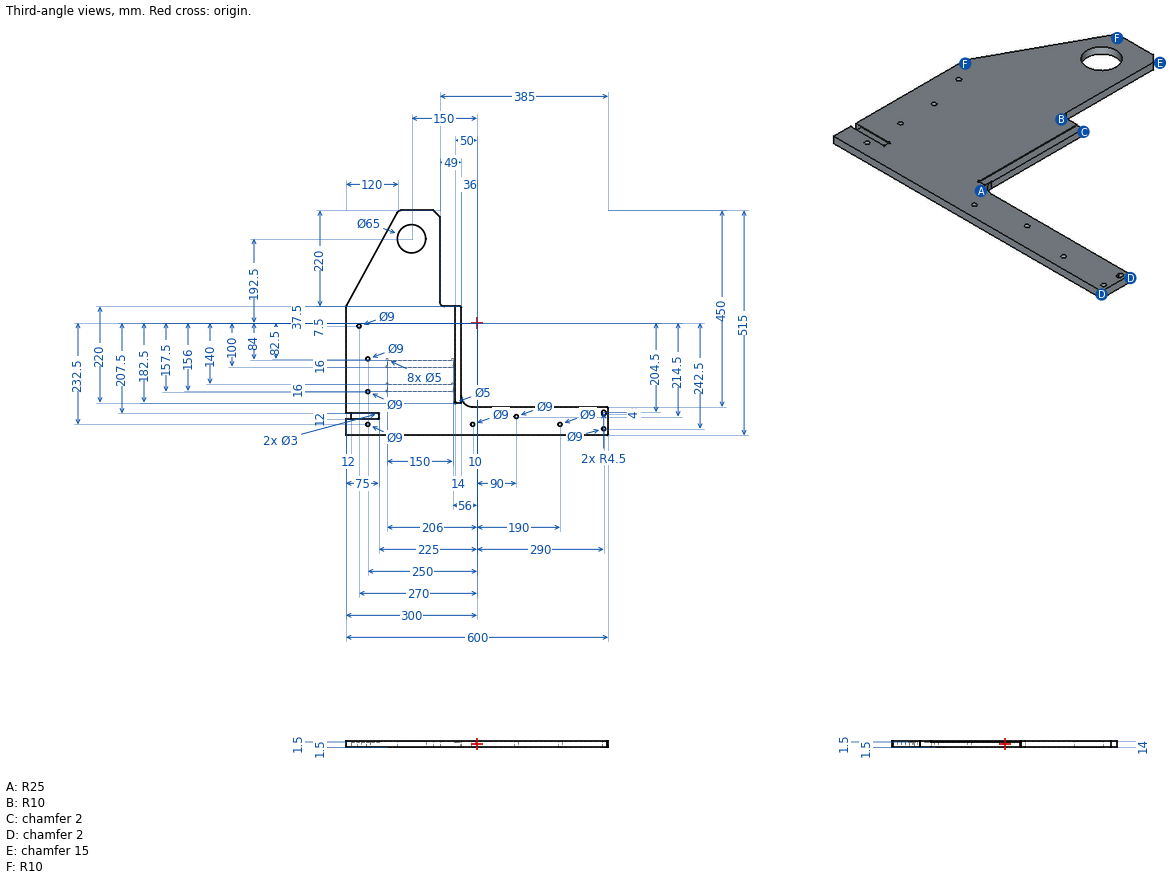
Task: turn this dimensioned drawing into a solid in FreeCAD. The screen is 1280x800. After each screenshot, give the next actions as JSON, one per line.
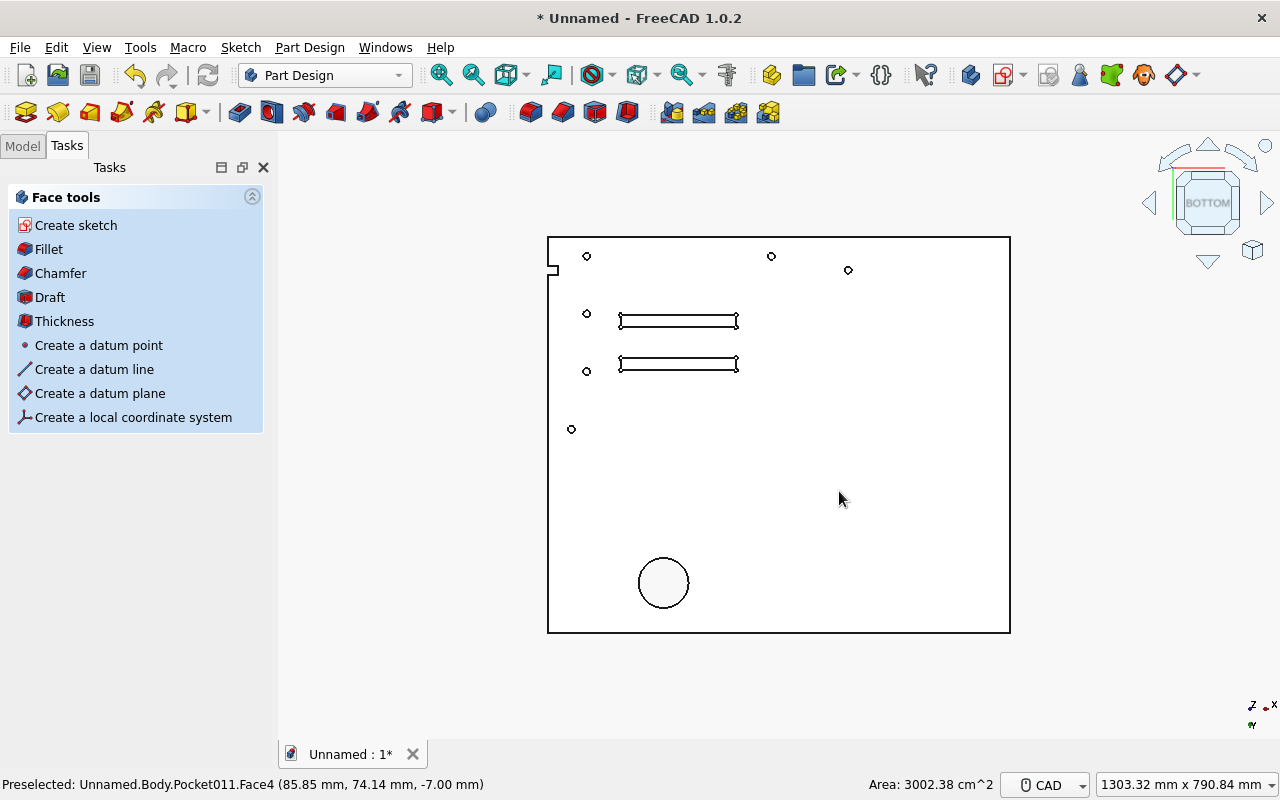
{"action": "left_click", "coordinate": [1004, 76]}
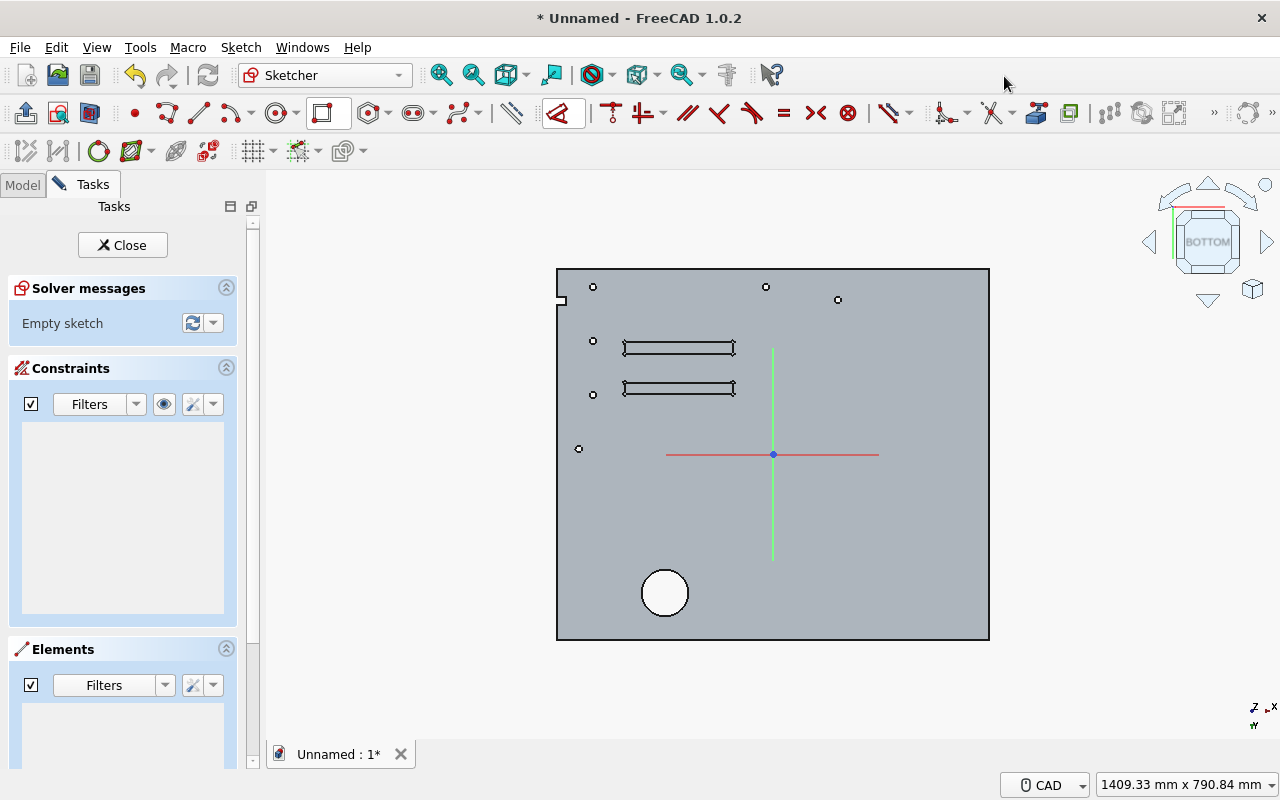
{"action": "scroll", "coordinate": [920, 278], "scroll_direction": "up", "scroll_amount": 15}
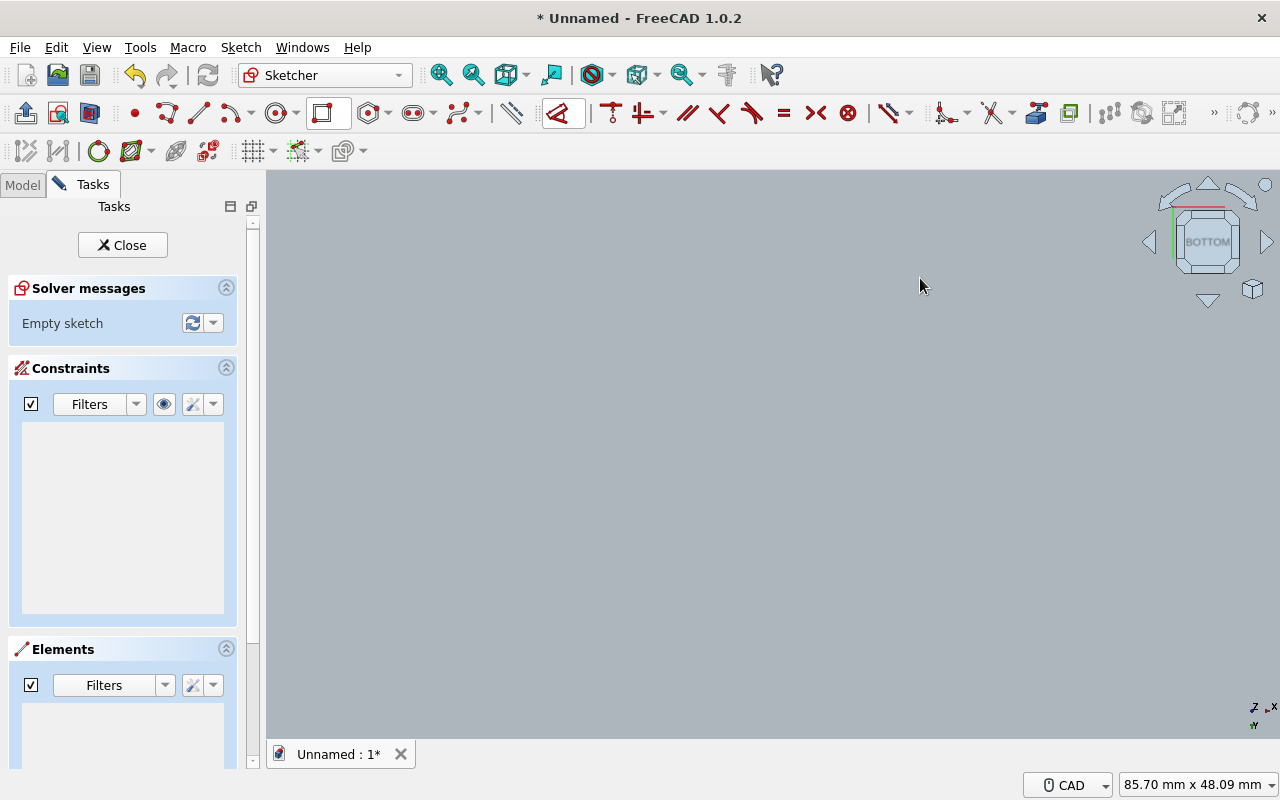
{"action": "scroll", "coordinate": [699, 462], "scroll_direction": "up", "scroll_amount": 5}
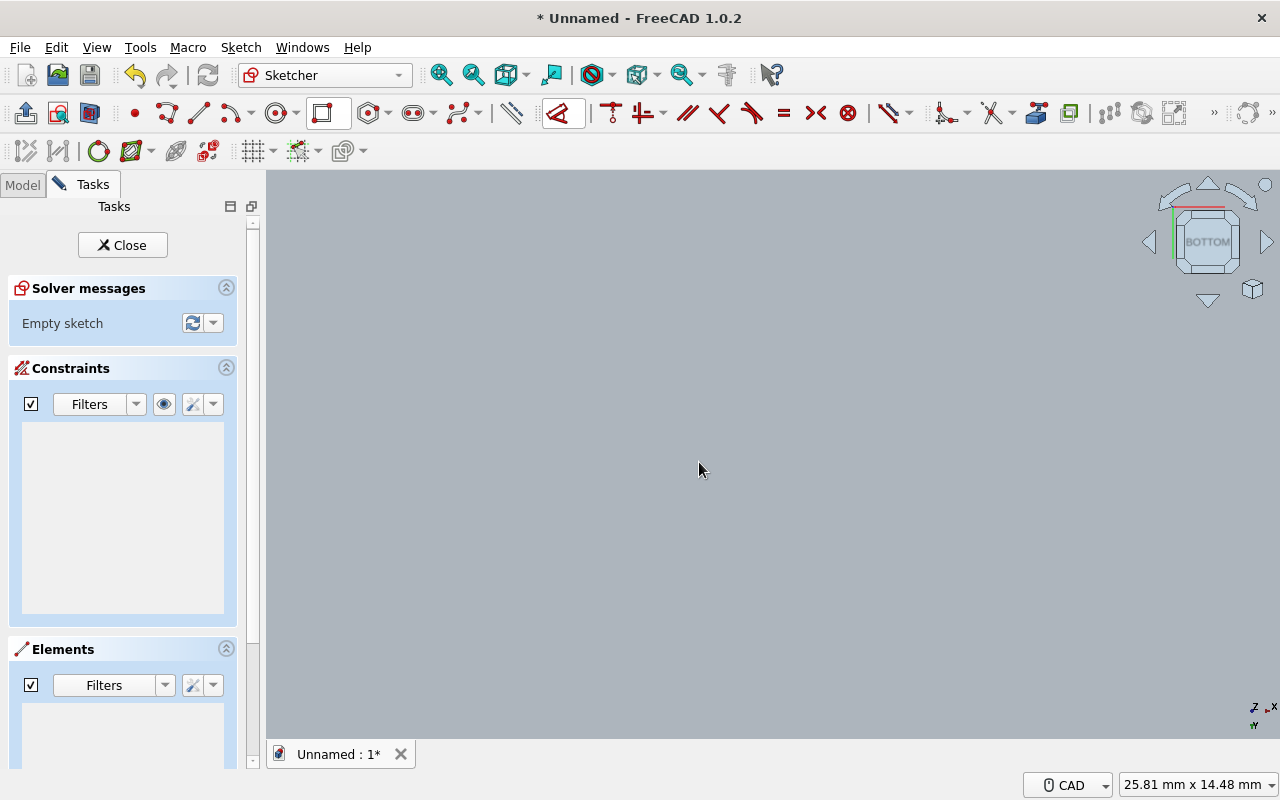
{"action": "left_click", "coordinate": [276, 114]}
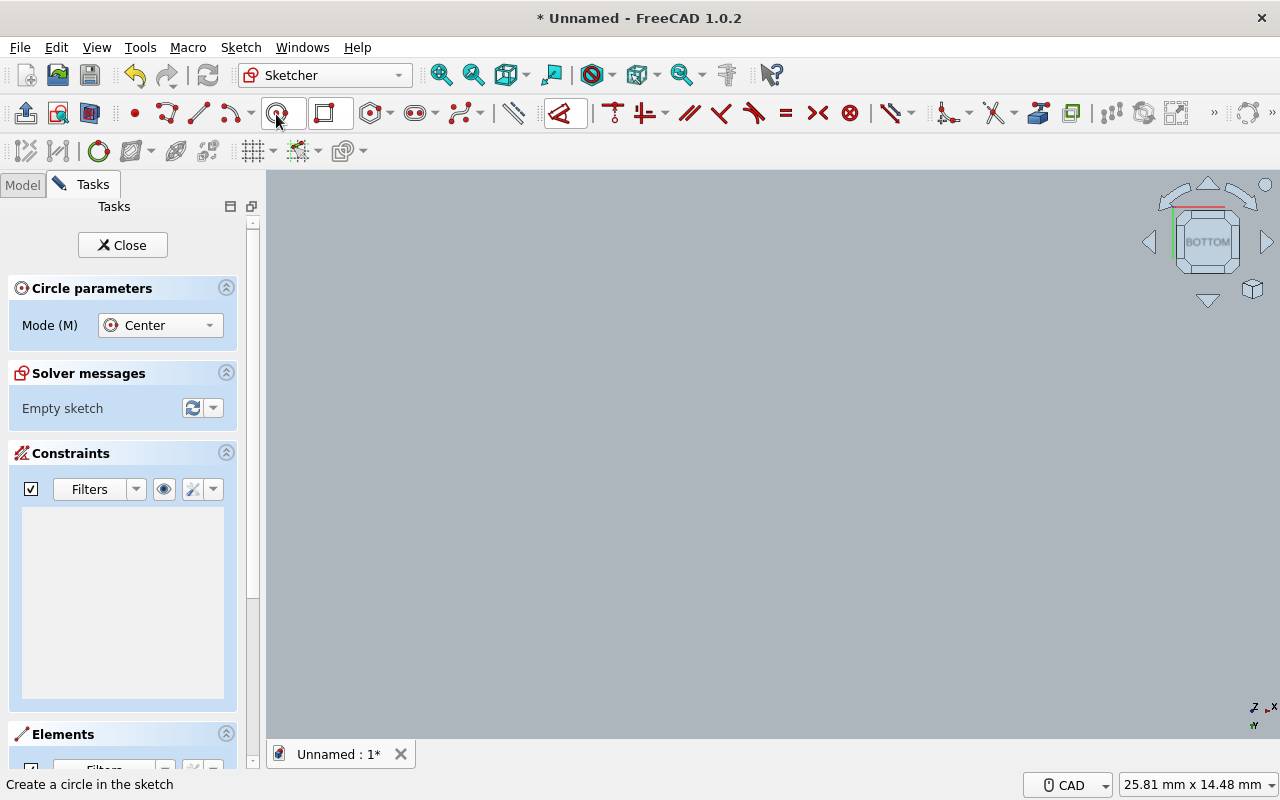
{"action": "left_click", "coordinate": [703, 454]}
{"action": "mouse_move", "coordinate": [828, 329]}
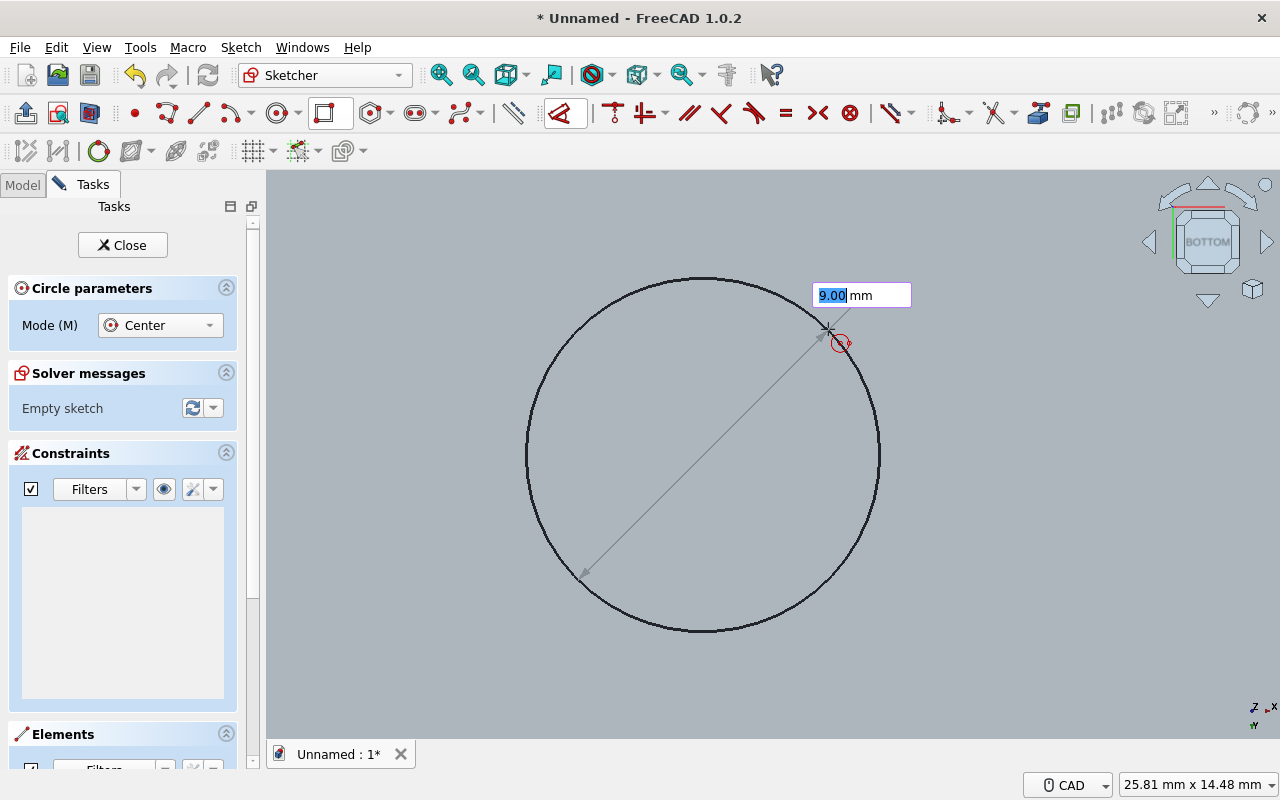
{"action": "type", "text": "9"}
{"action": "key", "text": "Return"}
{"action": "key", "text": "Escape"}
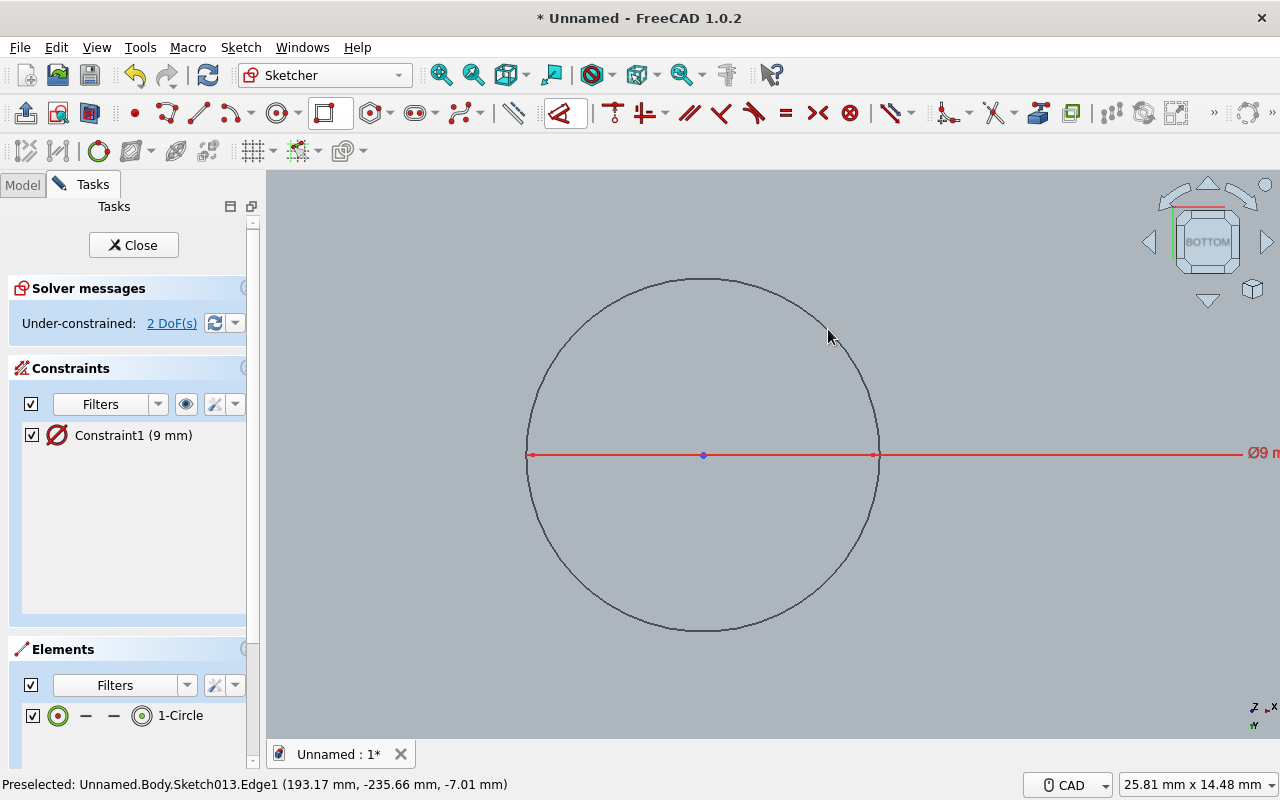
{"action": "left_click", "coordinate": [703, 455]}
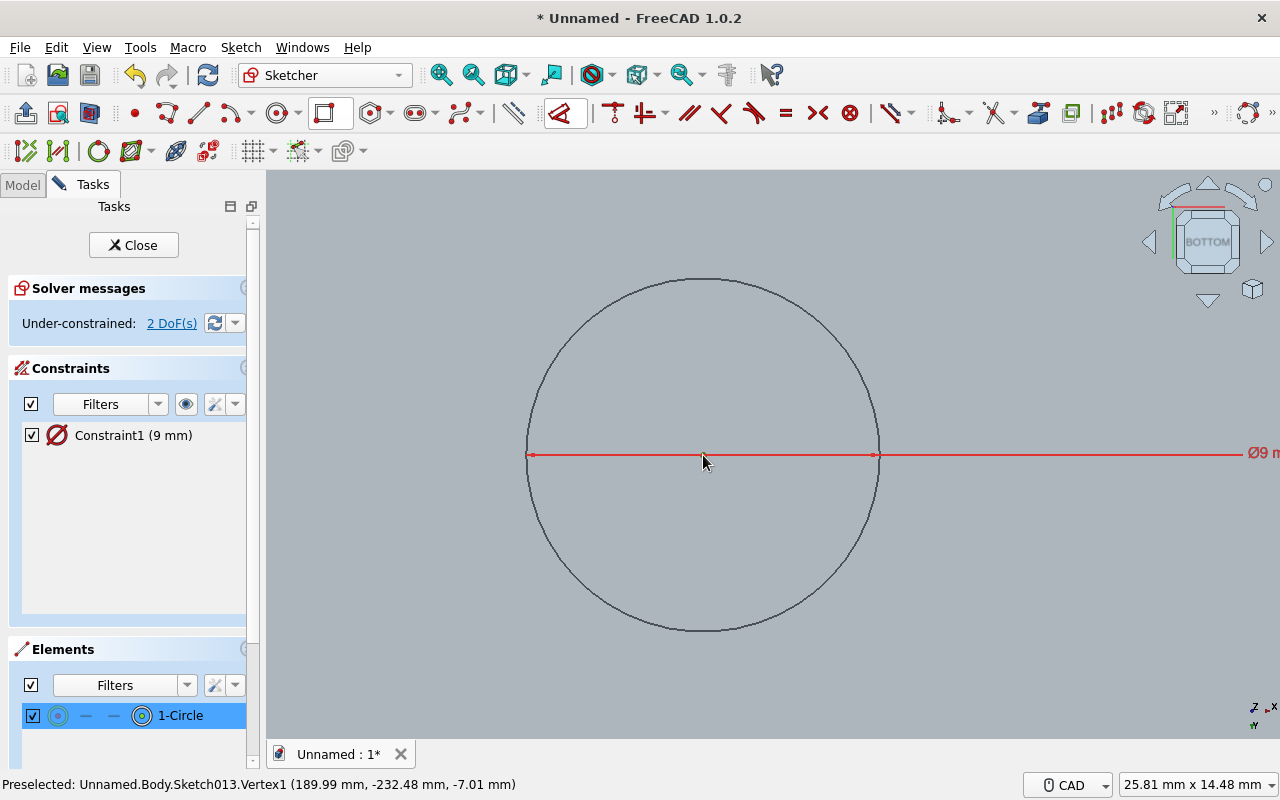
{"action": "left_click", "coordinate": [582, 114]}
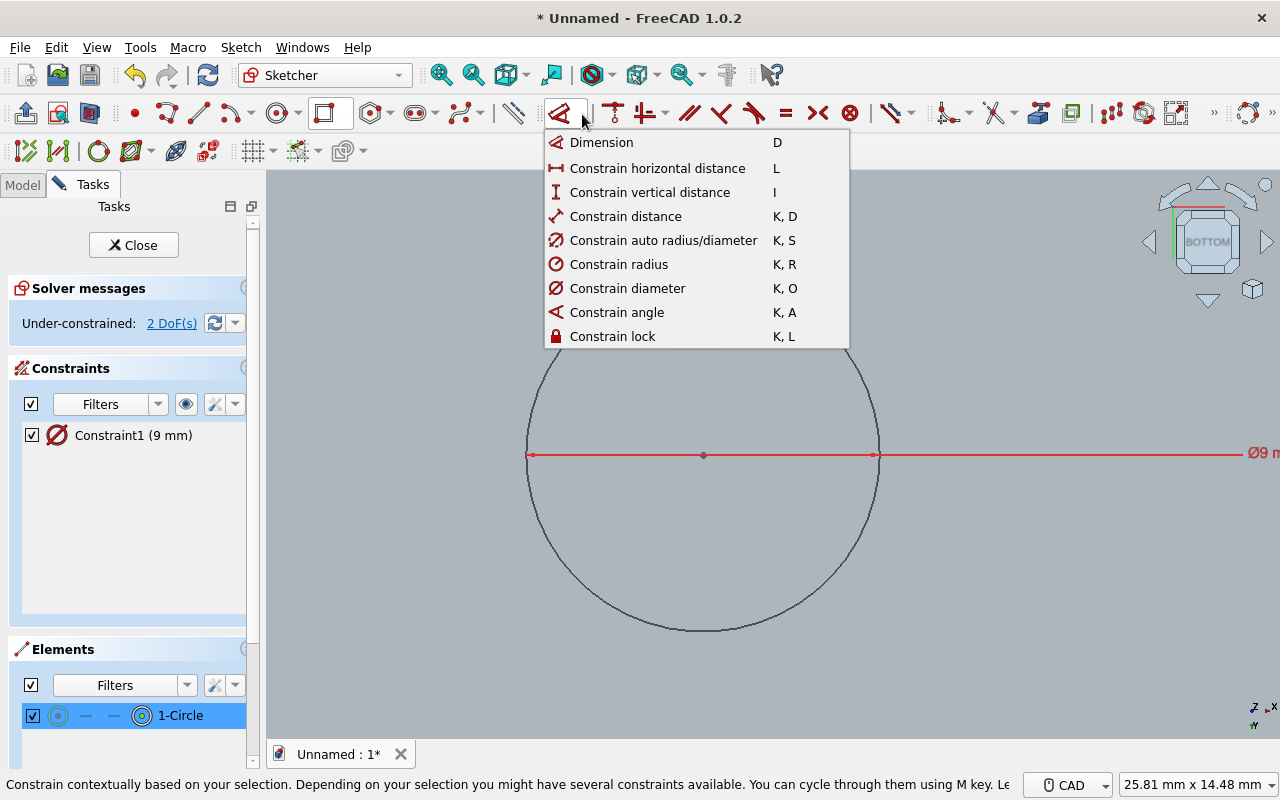
{"action": "left_click", "coordinate": [697, 168]}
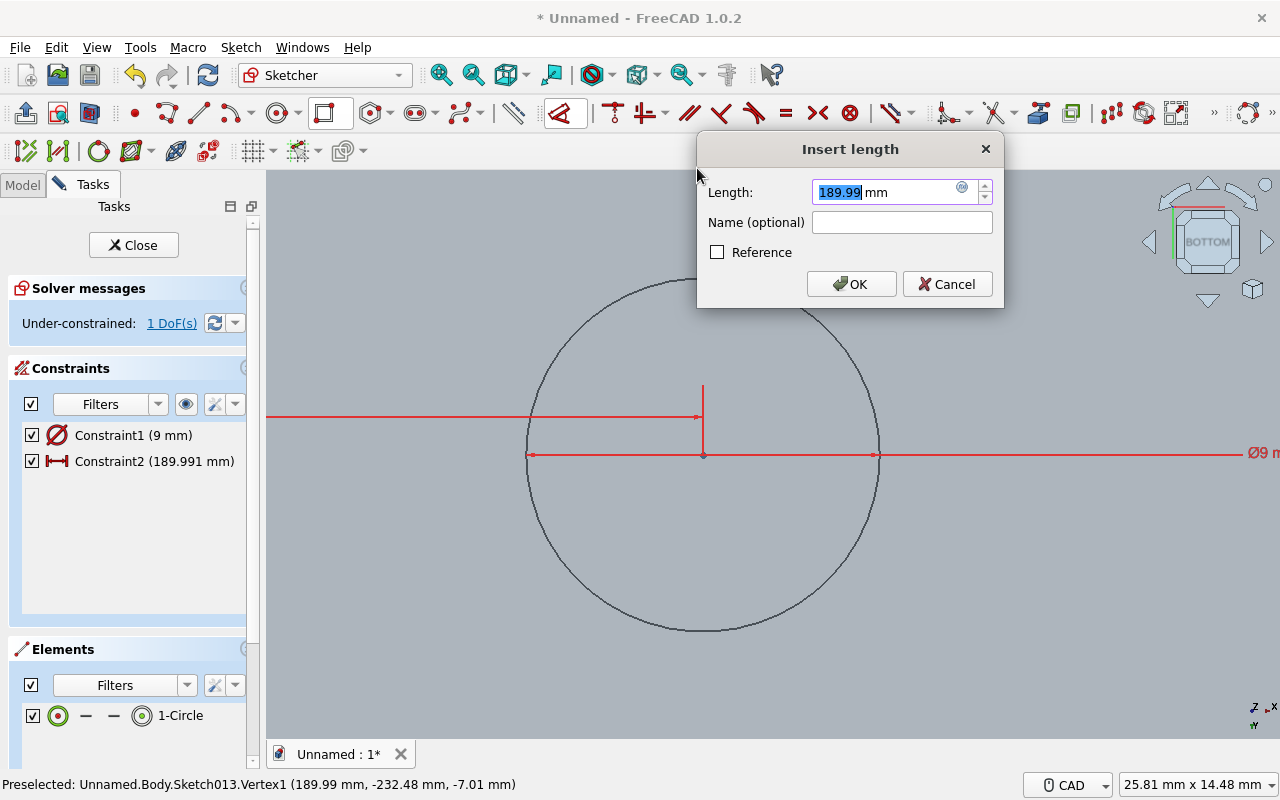
{"action": "type", "text": "190"}
{"action": "key", "text": "Return"}